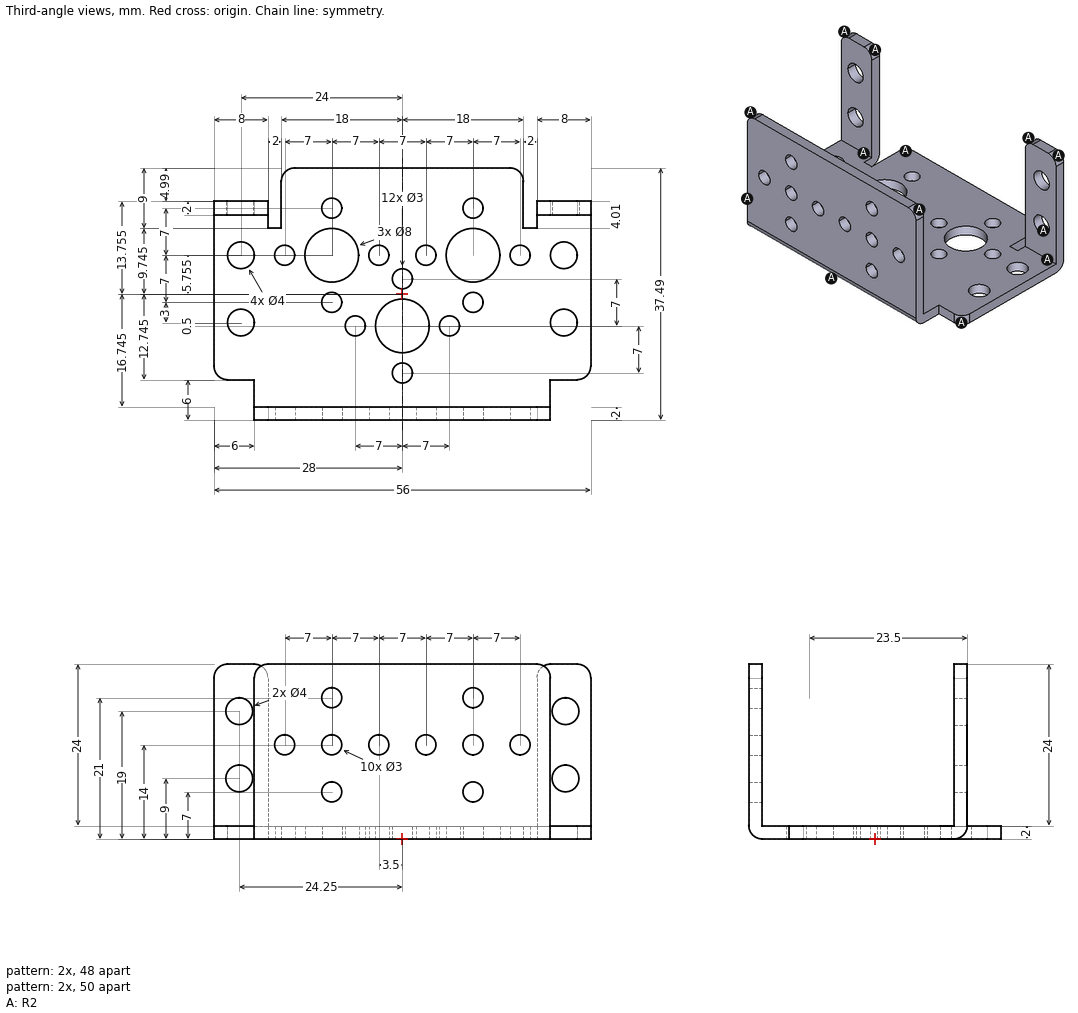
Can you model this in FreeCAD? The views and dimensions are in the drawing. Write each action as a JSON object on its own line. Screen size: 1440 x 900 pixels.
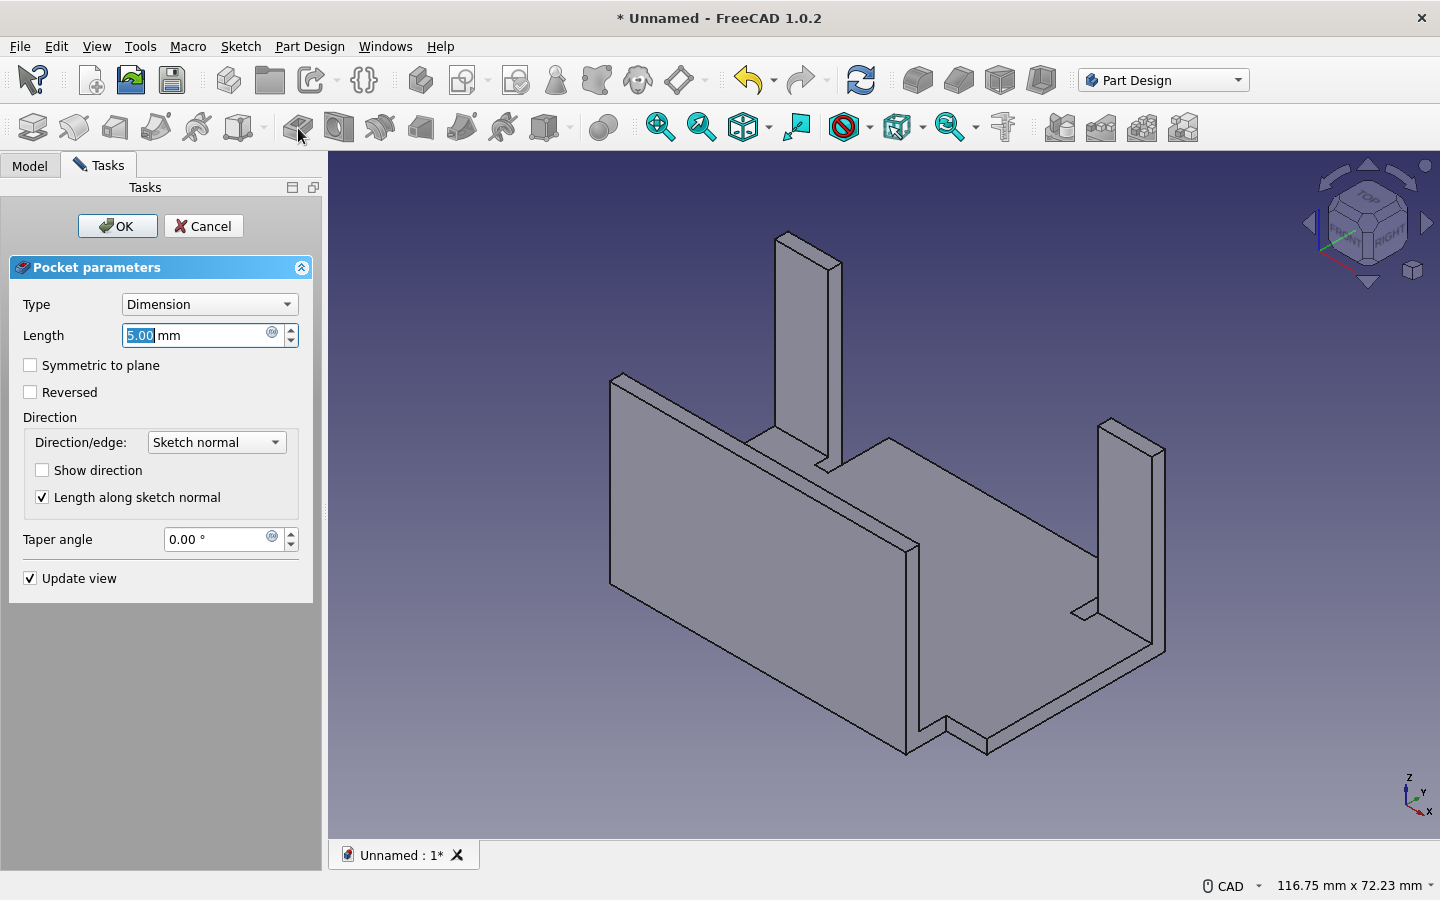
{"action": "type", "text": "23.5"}
{"action": "key", "text": "Tab"}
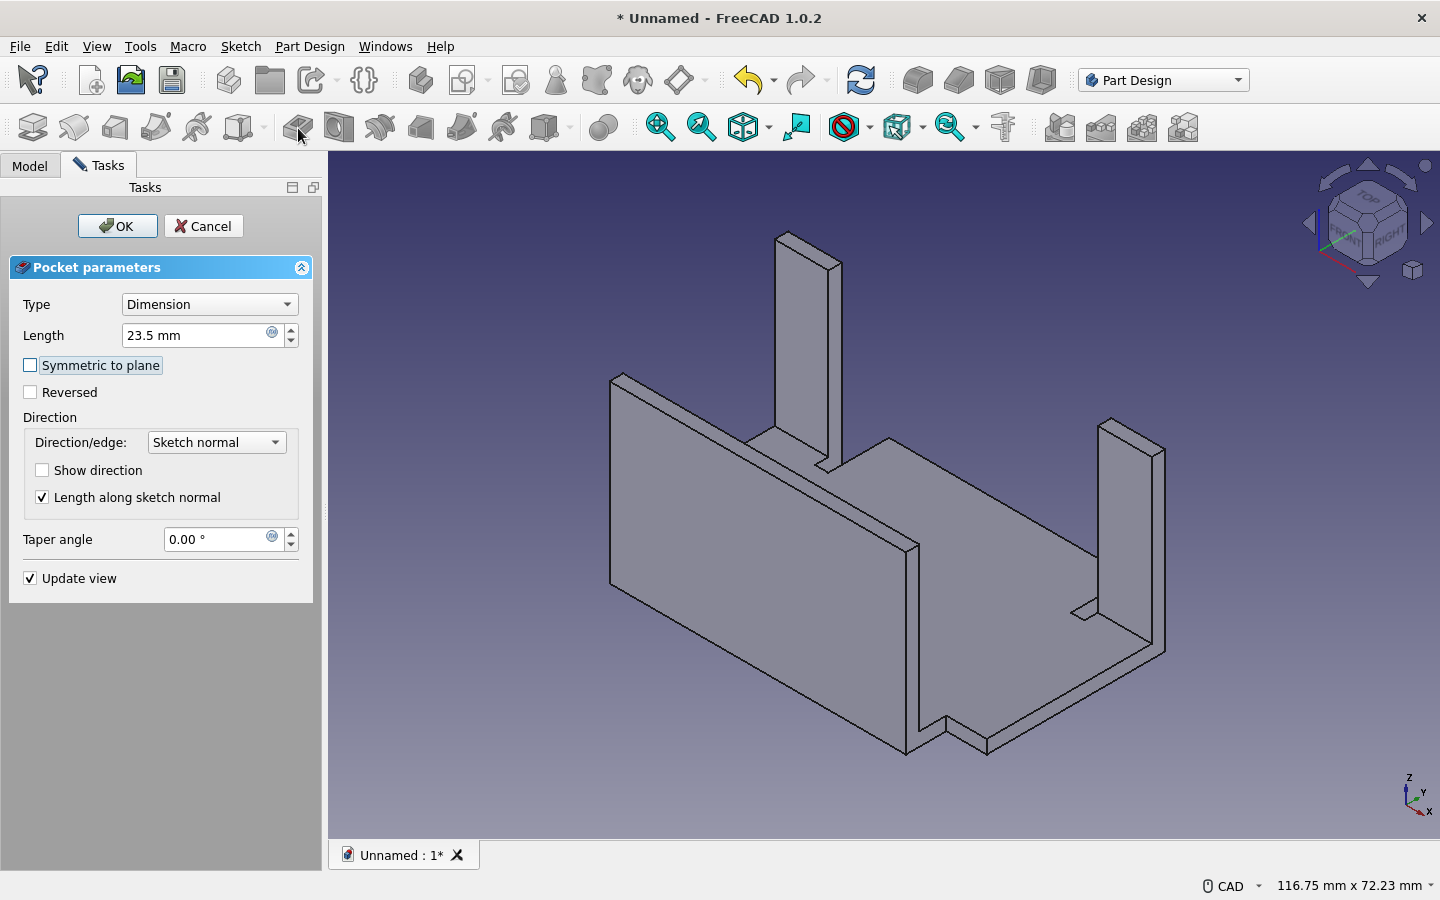
{"action": "left_click", "coordinate": [118, 226]}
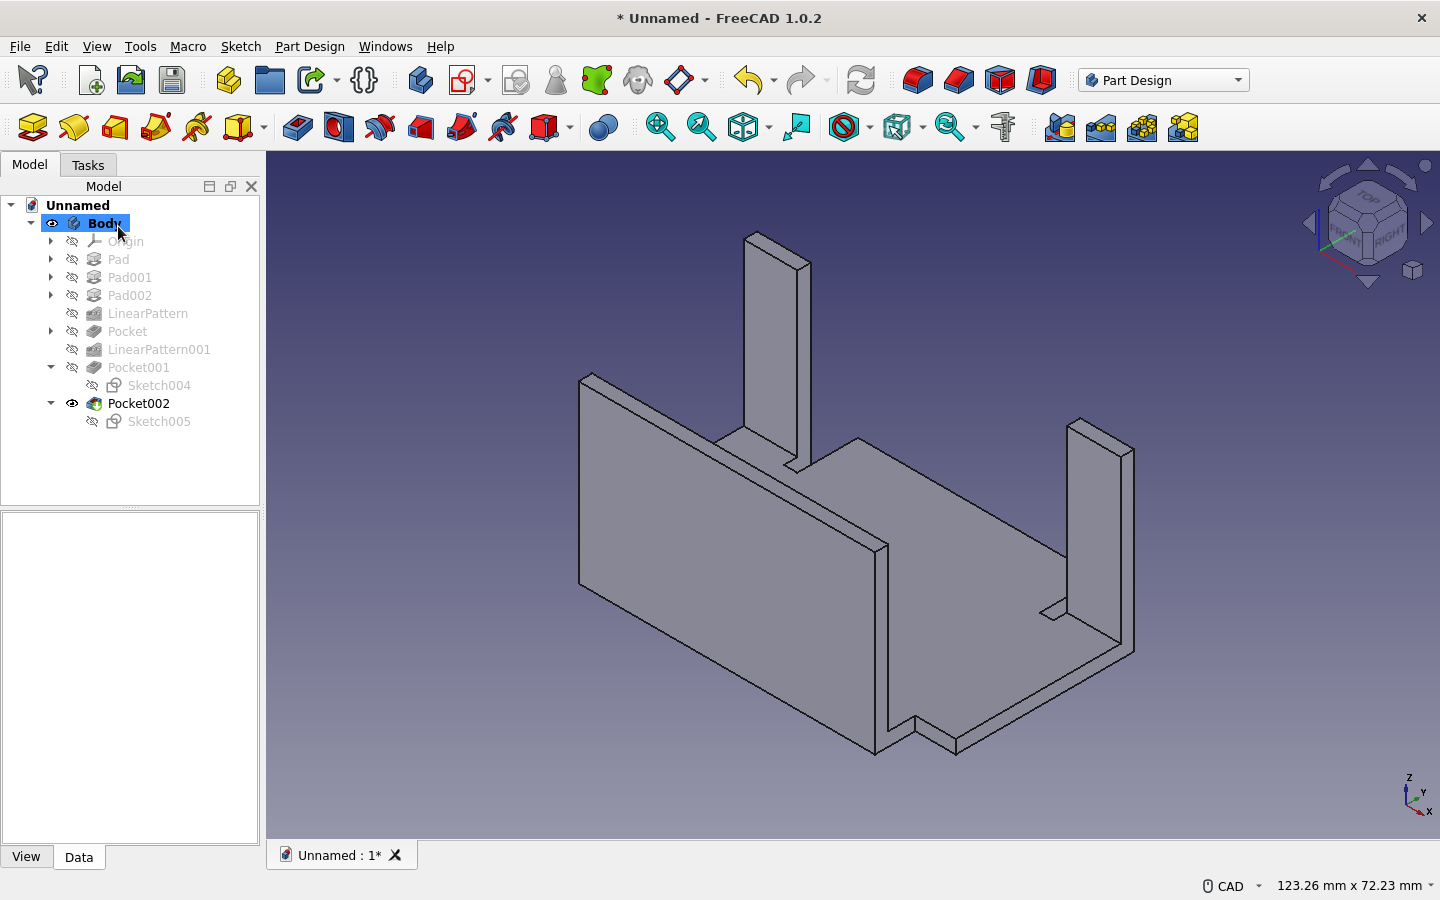
{"action": "left_click", "coordinate": [914, 607]}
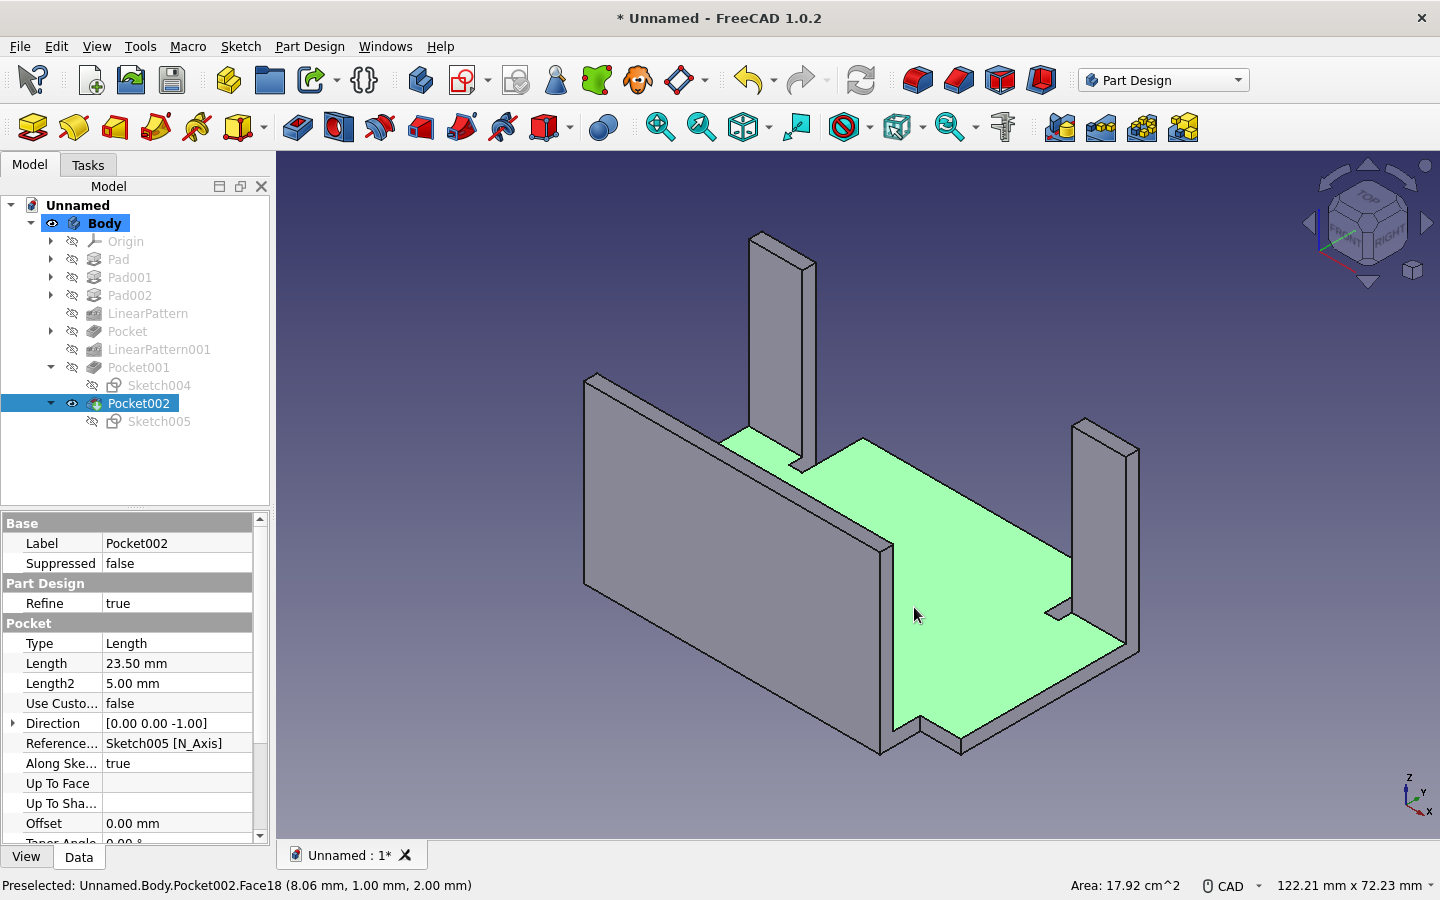
{"action": "left_click", "coordinate": [462, 80]}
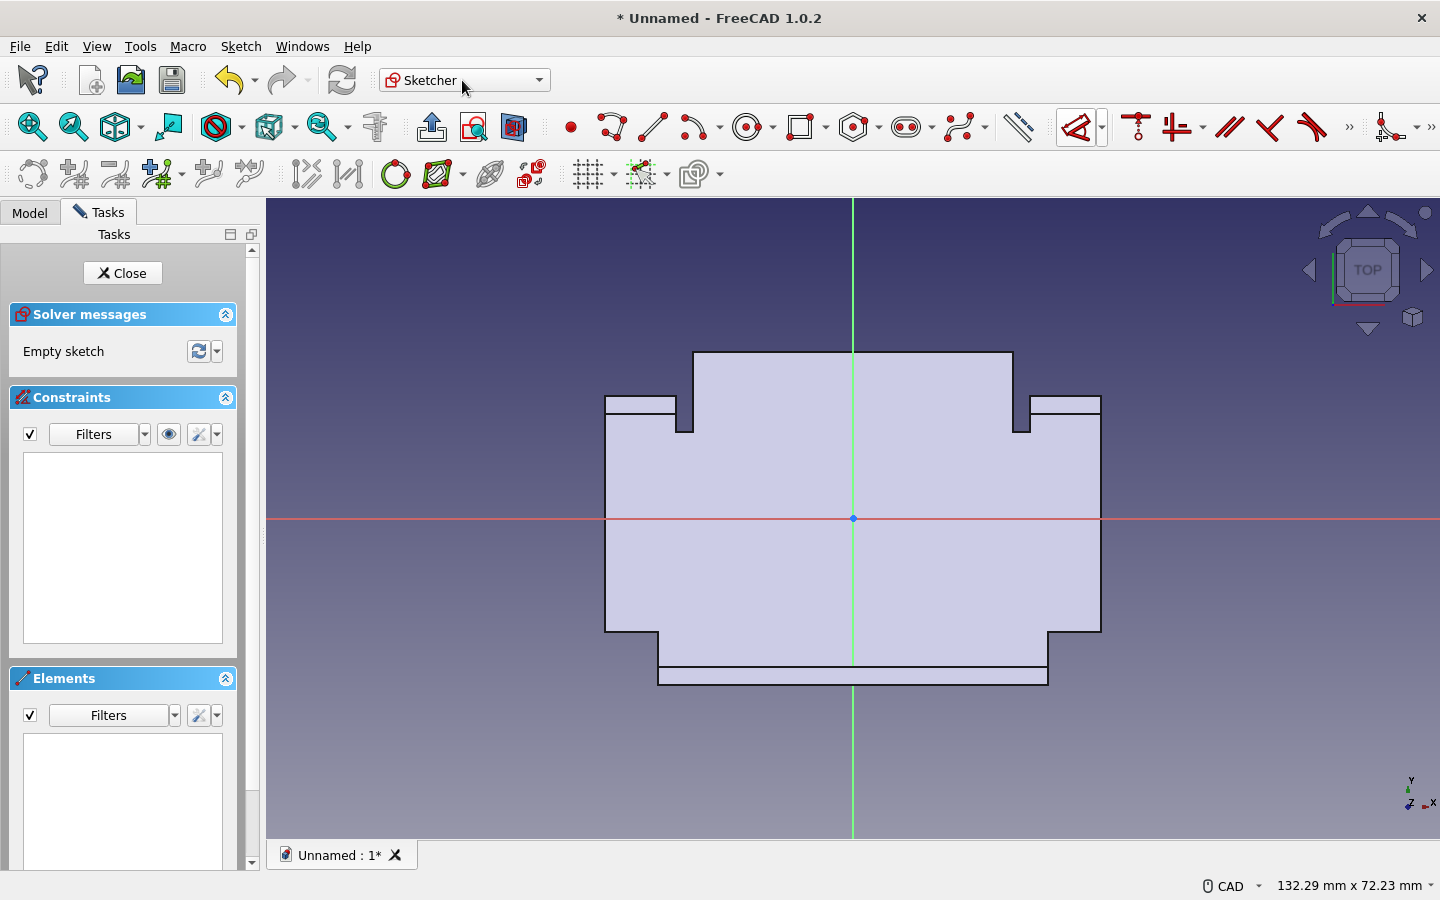
{"action": "key", "text": "q s"}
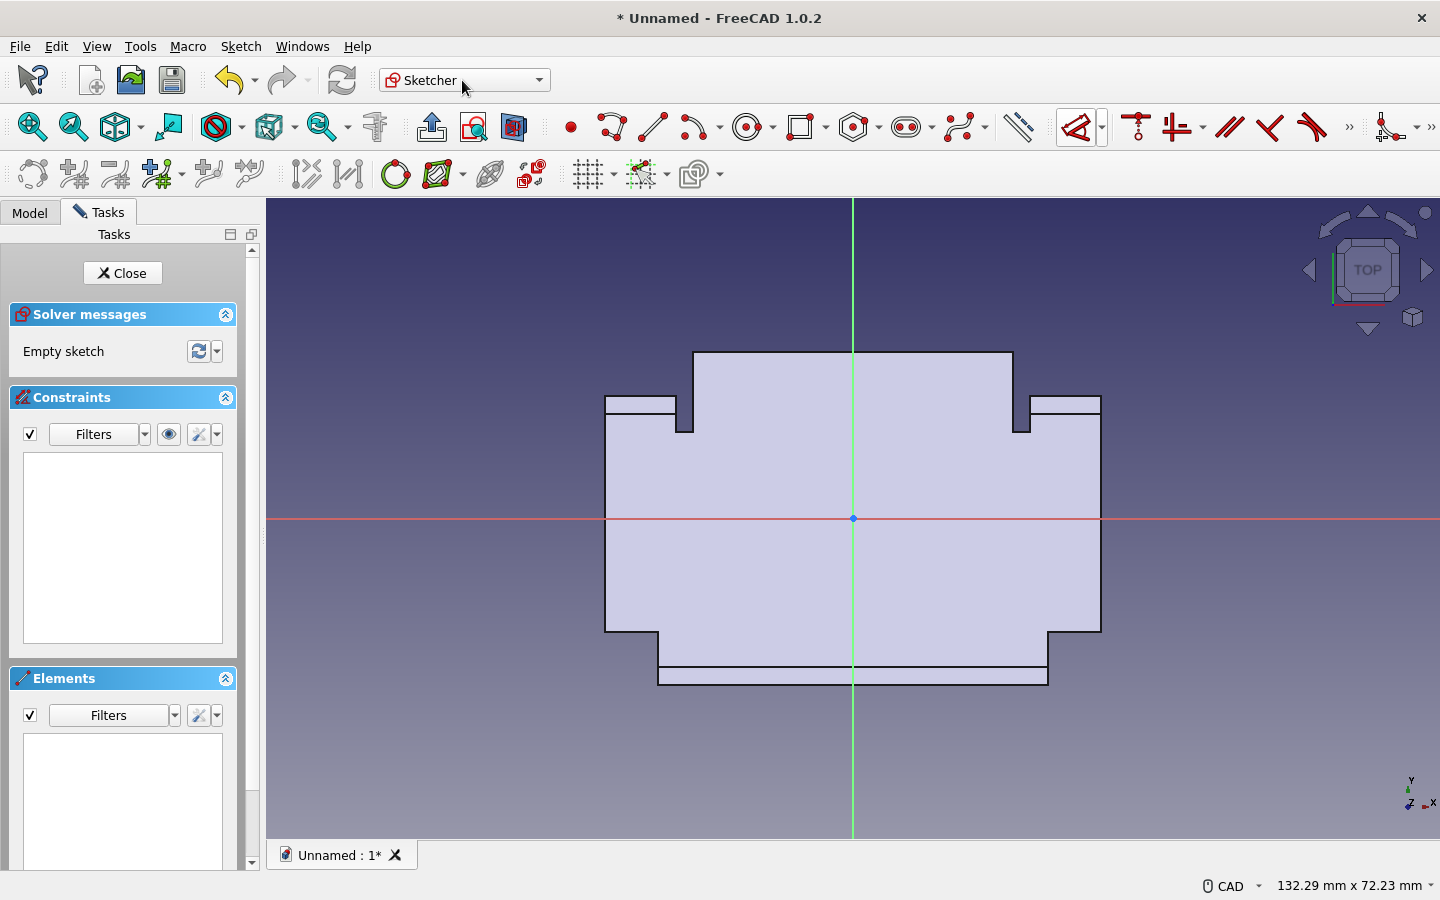
{"action": "scroll", "coordinate": [992, 505], "scroll_direction": "up", "scroll_amount": 2}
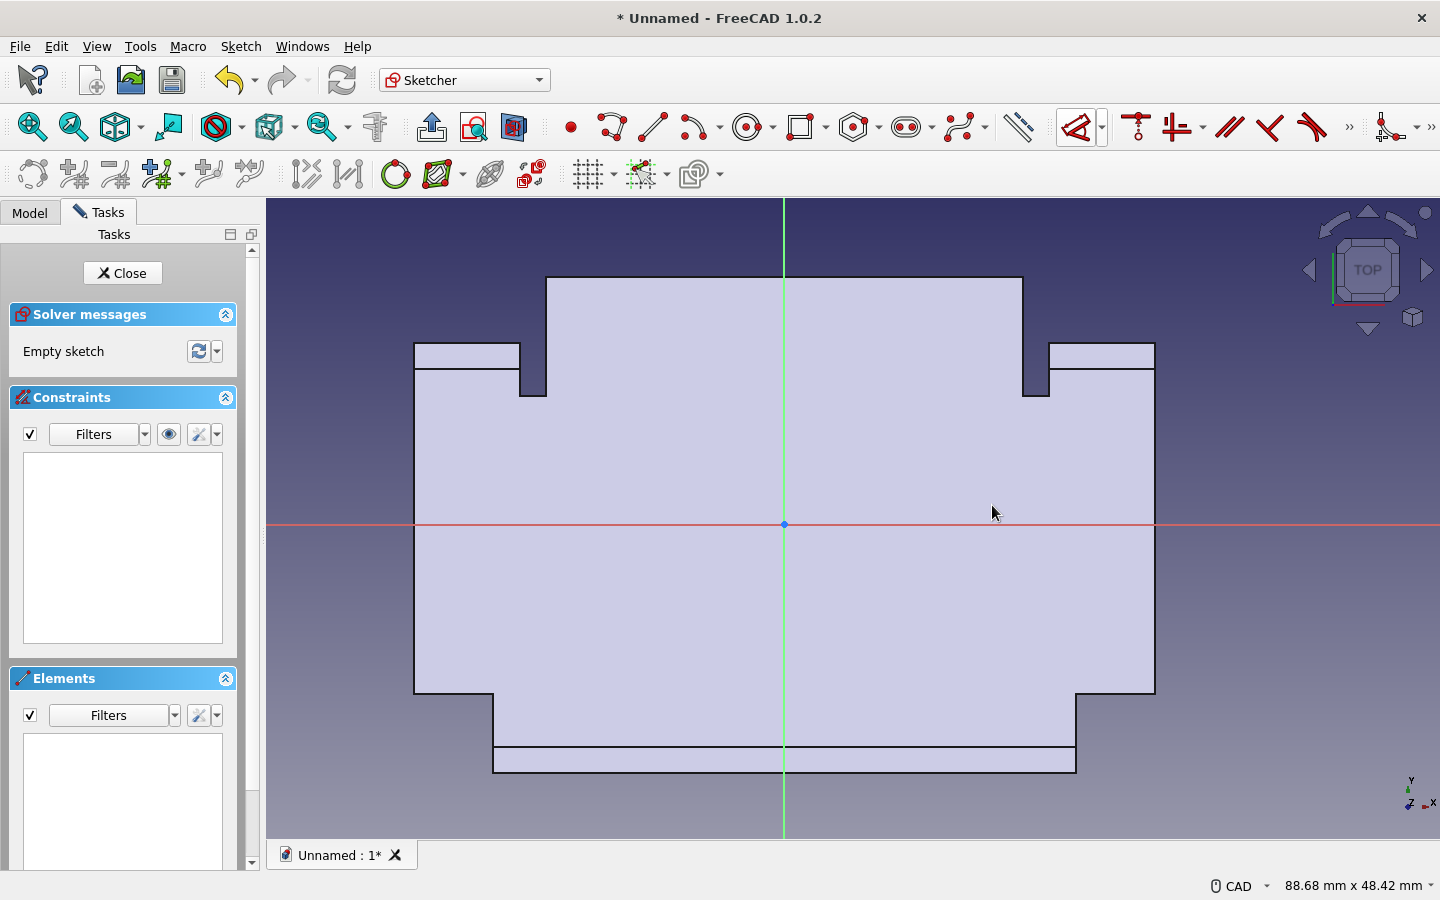
{"action": "key", "text": "g c"}